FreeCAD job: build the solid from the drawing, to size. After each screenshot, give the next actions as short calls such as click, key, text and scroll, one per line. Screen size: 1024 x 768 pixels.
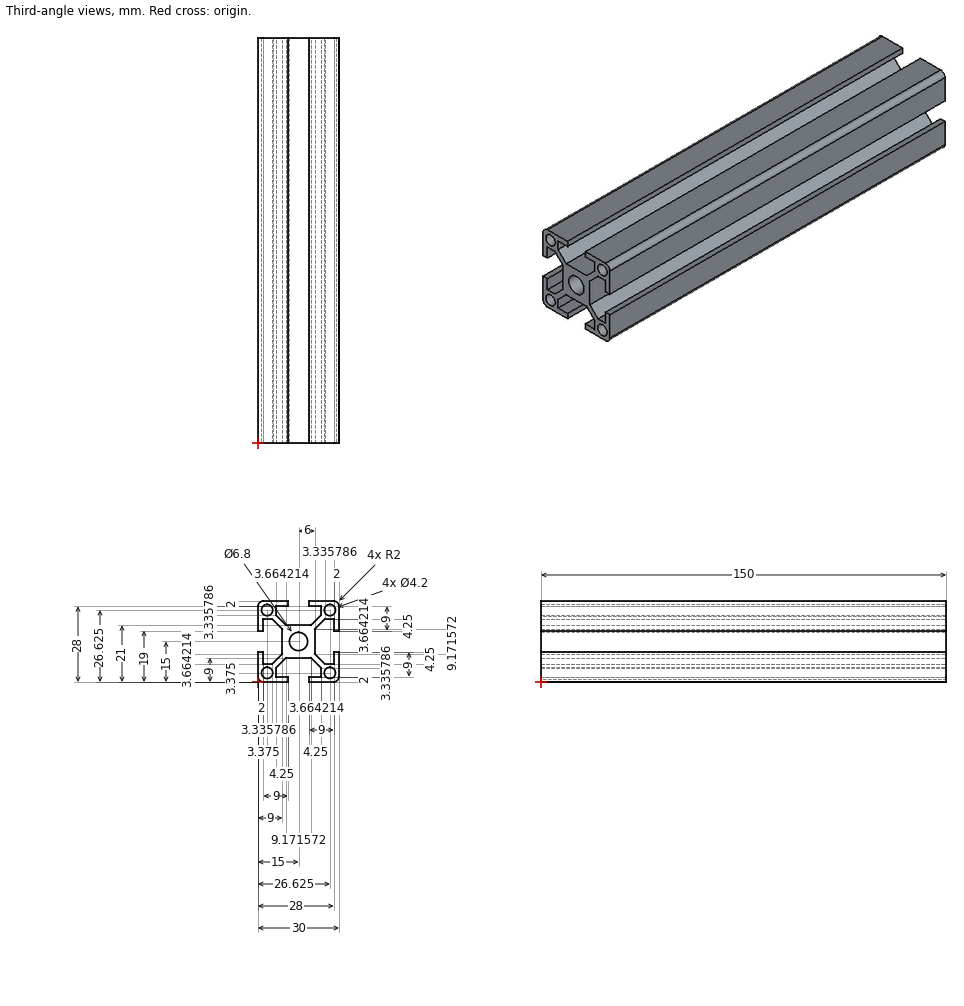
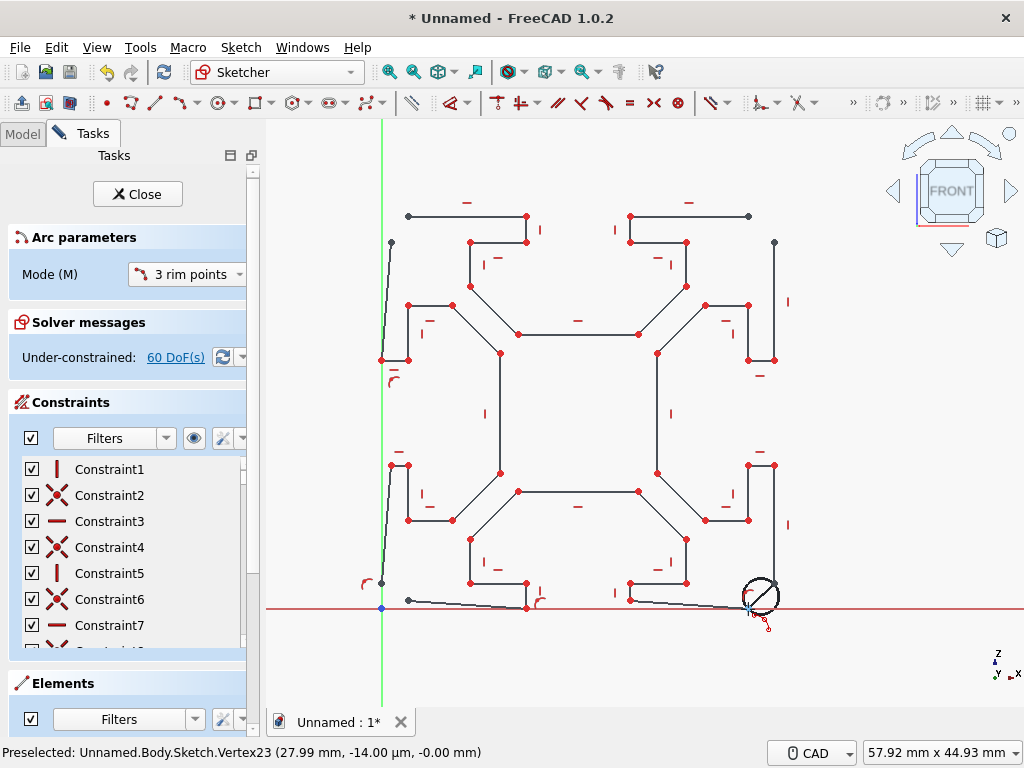
scroll(767, 601, up, 4)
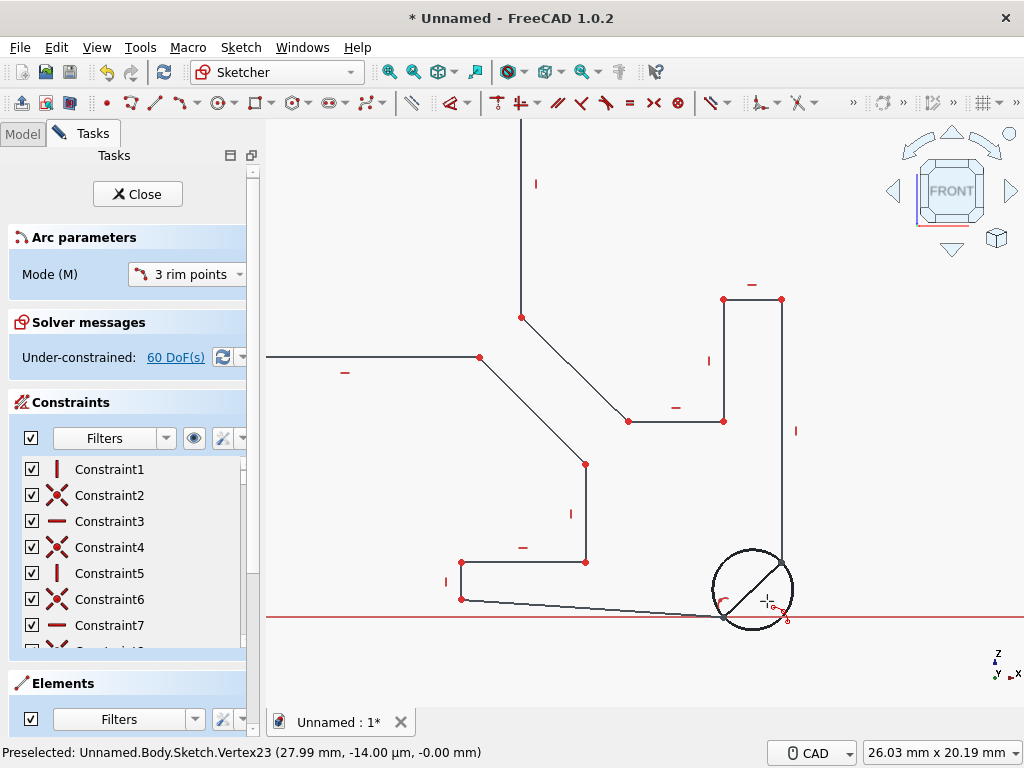
click(766, 600)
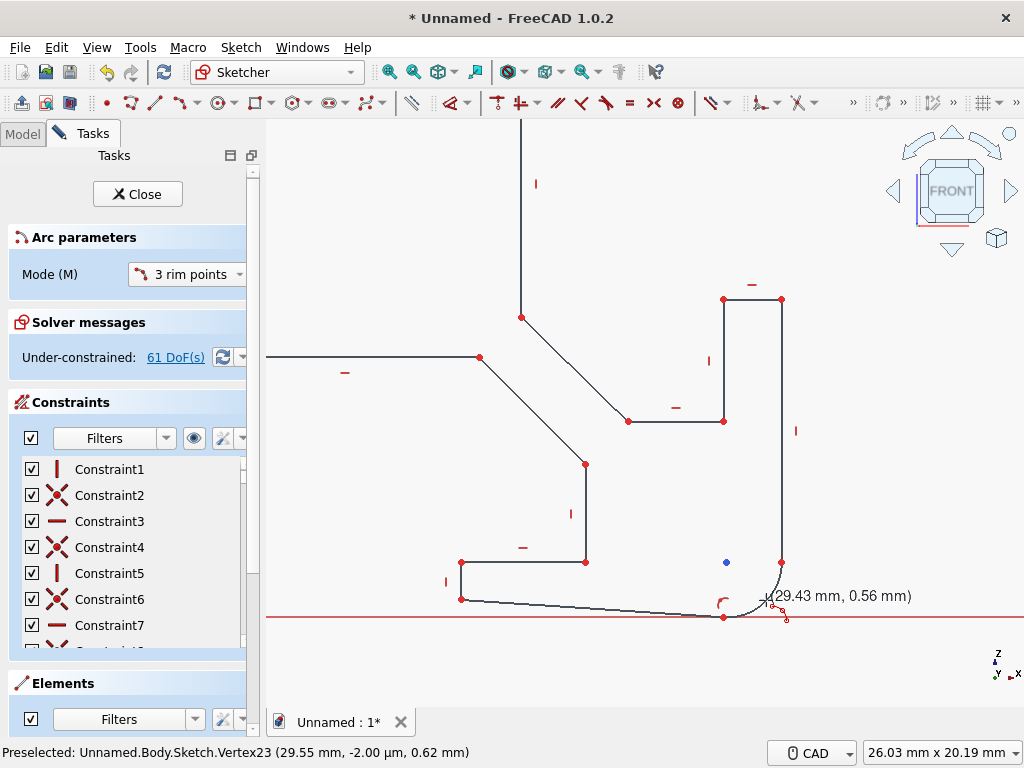
scroll(765, 603, down, 4)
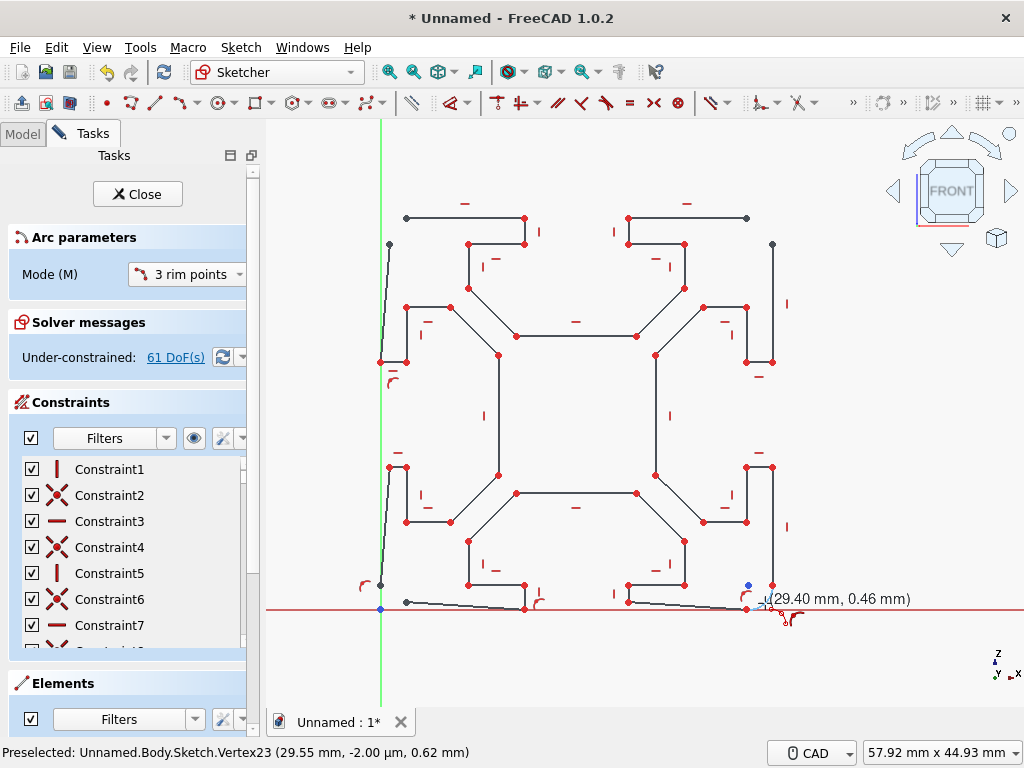
click(407, 602)
click(381, 585)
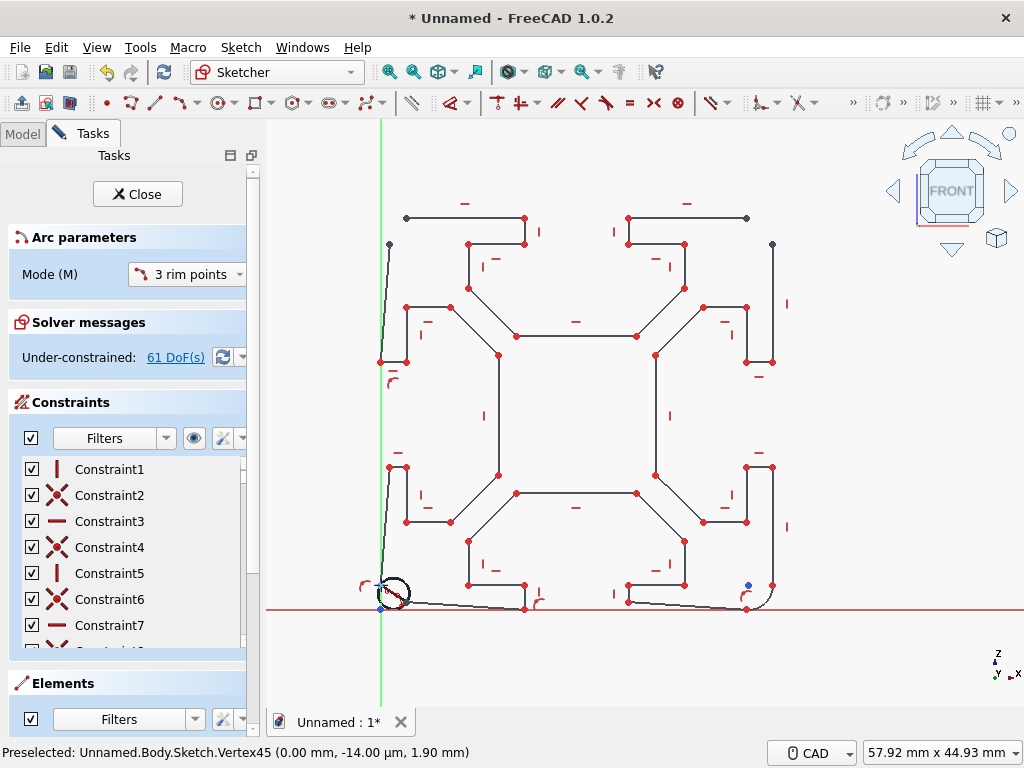
scroll(388, 602, up, 4)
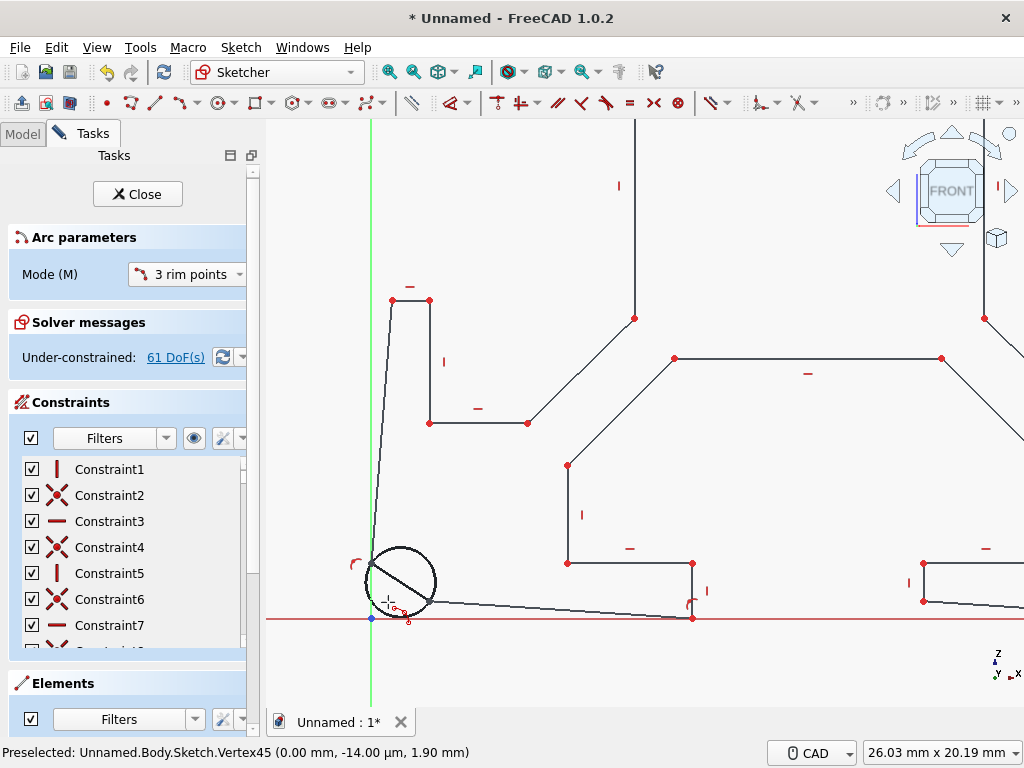
click(389, 602)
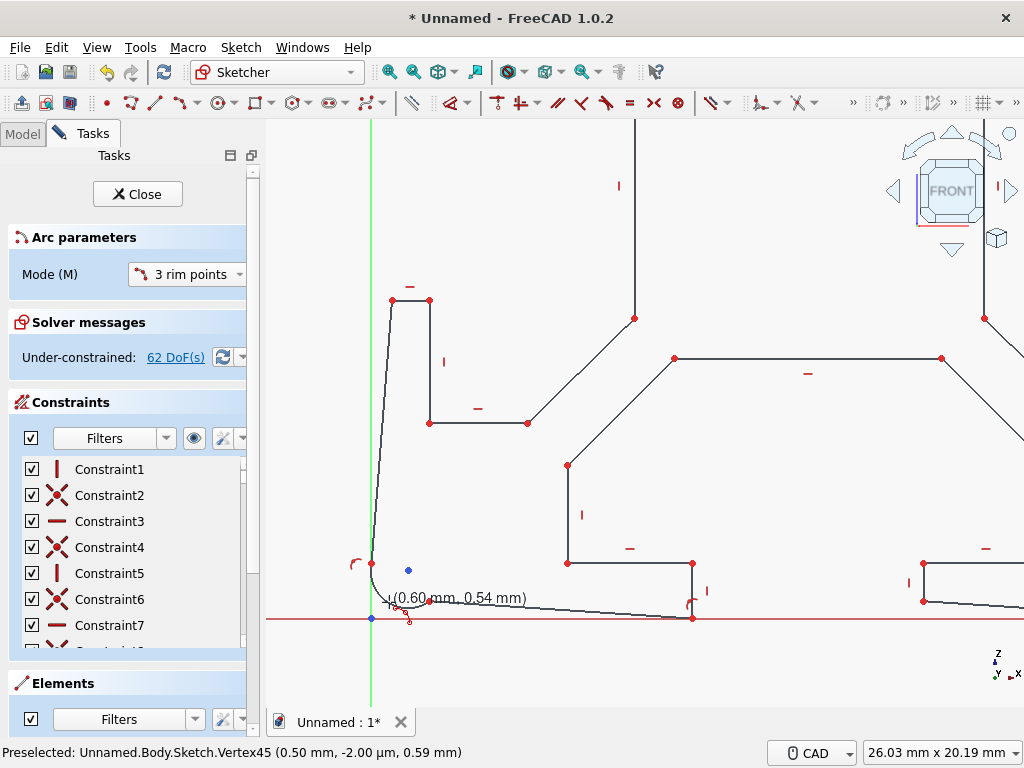
scroll(387, 602, down, 4)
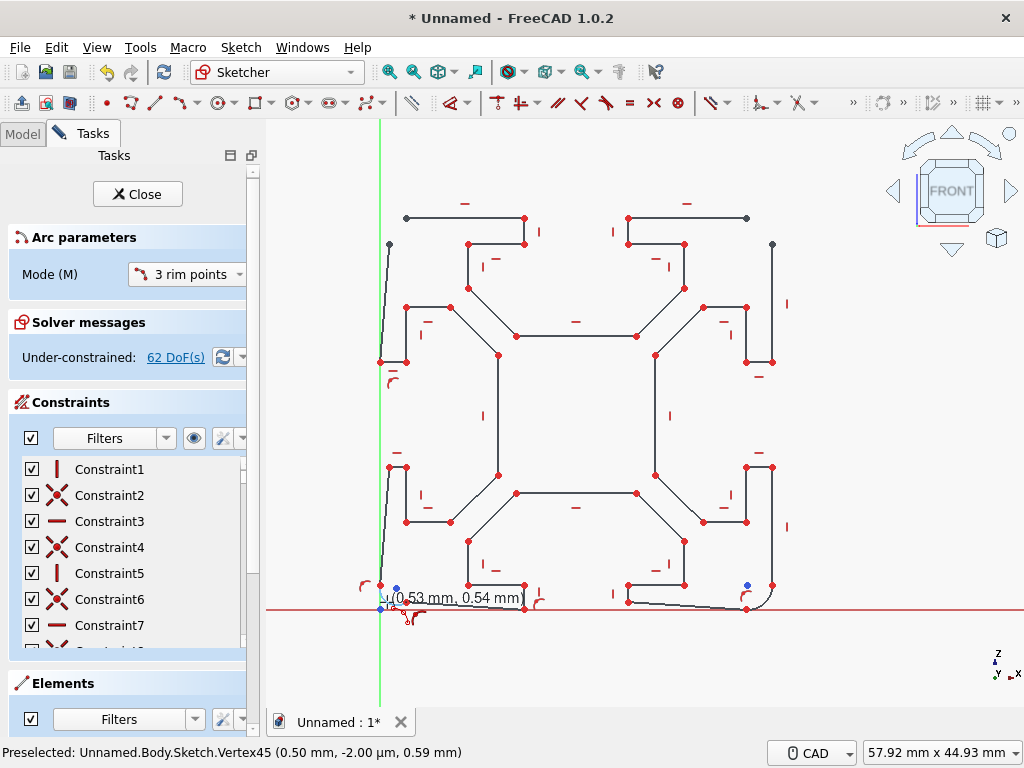
click(389, 244)
click(406, 218)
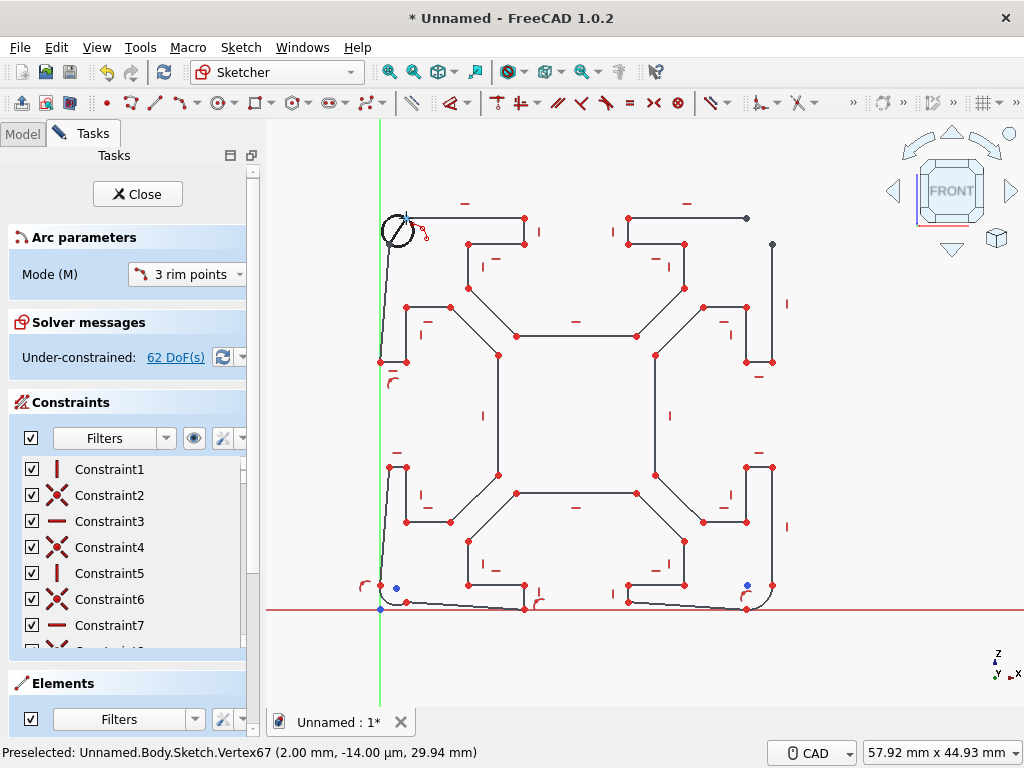
scroll(388, 225, up, 4)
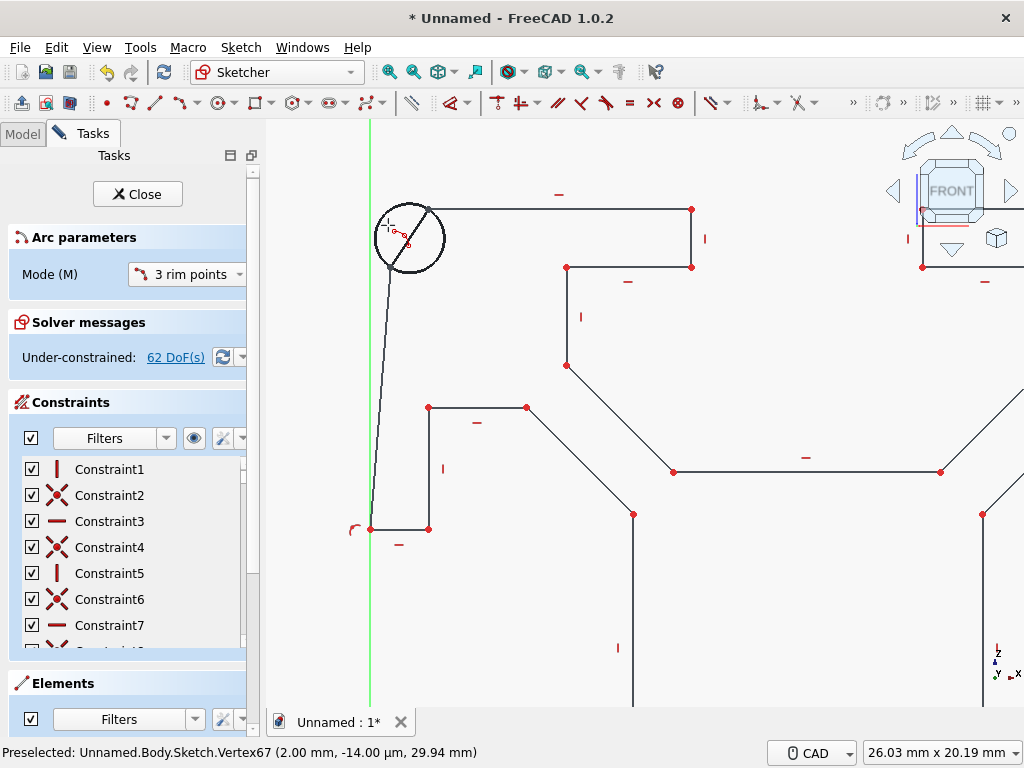
click(387, 225)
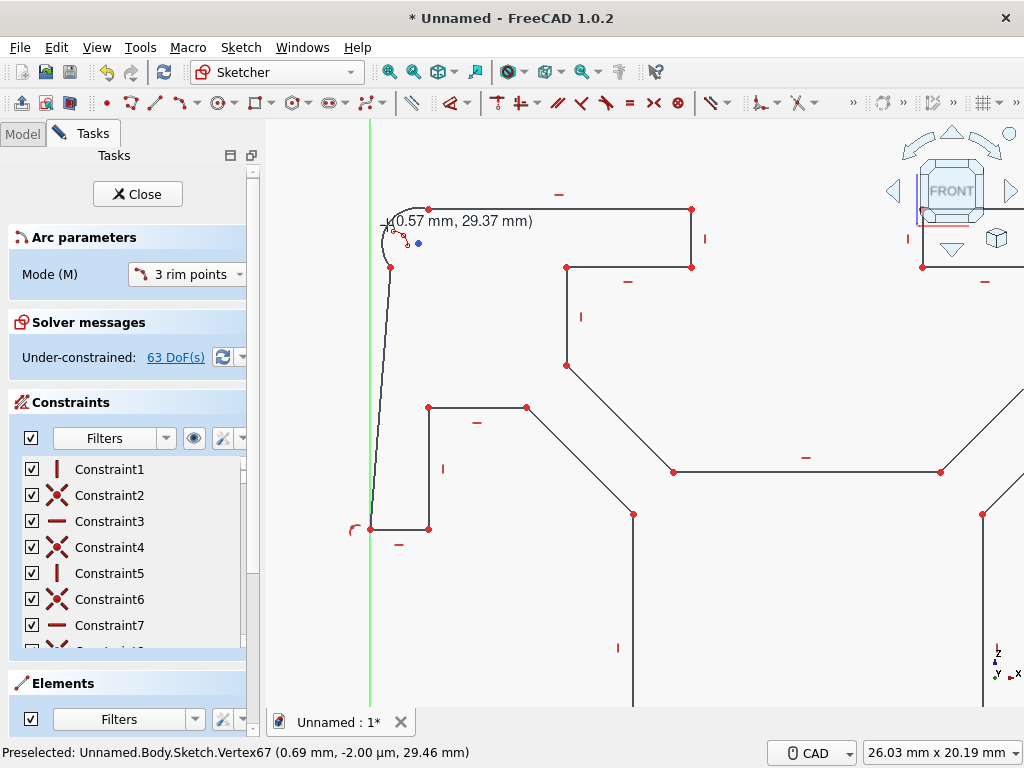
scroll(388, 224, down, 4)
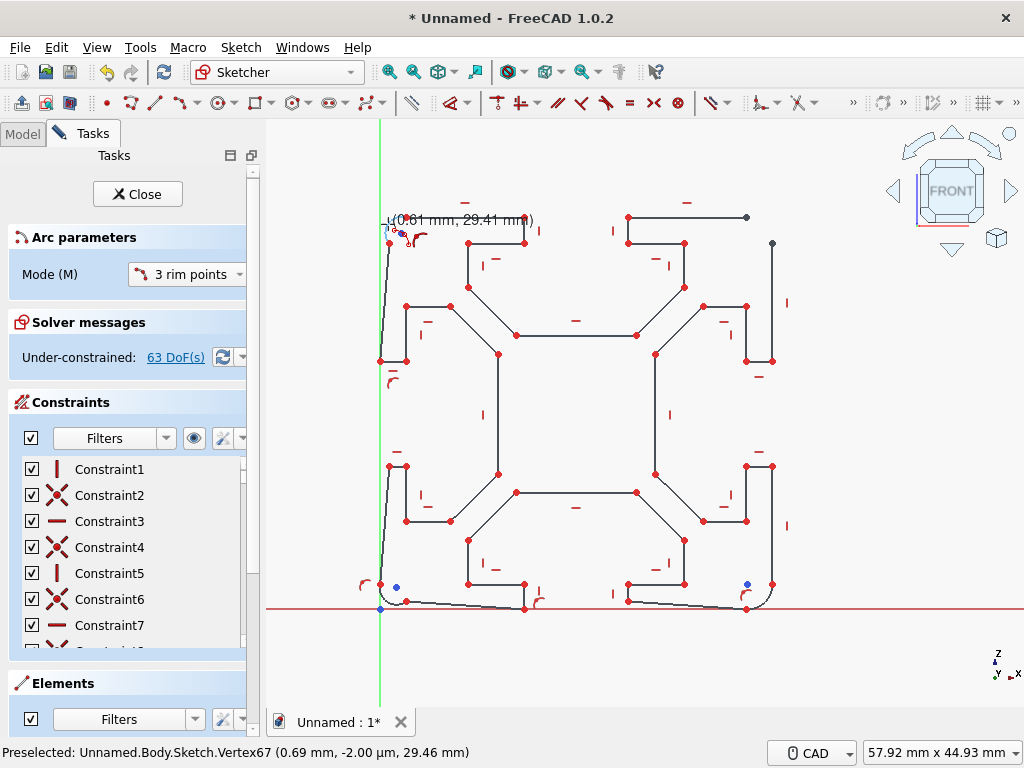
click(746, 218)
click(772, 244)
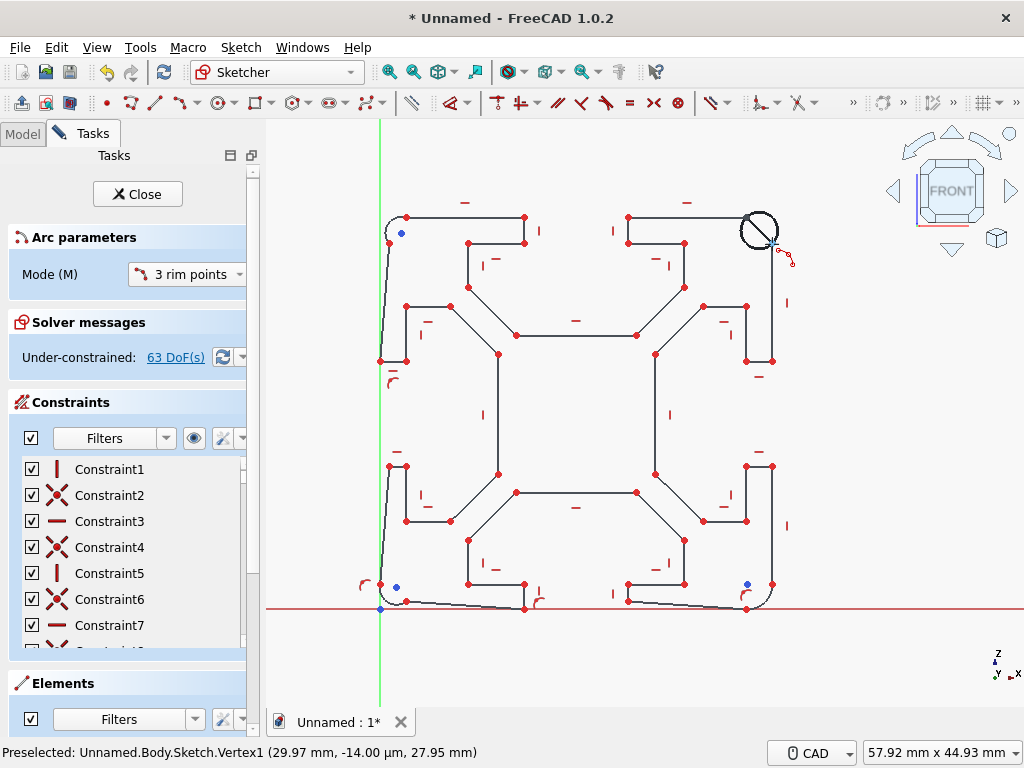
scroll(765, 224, up, 4)